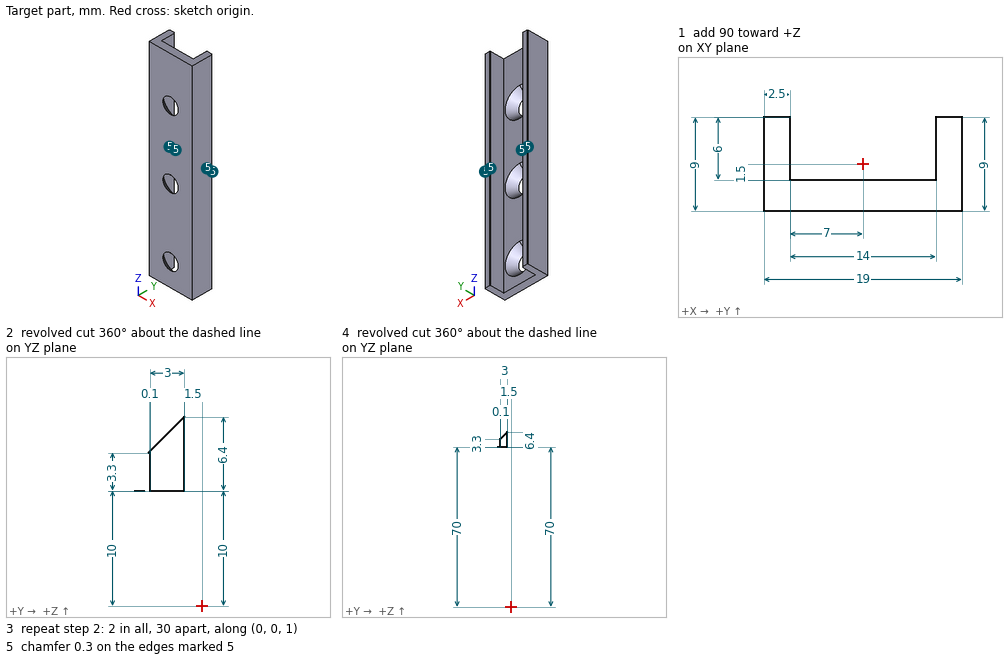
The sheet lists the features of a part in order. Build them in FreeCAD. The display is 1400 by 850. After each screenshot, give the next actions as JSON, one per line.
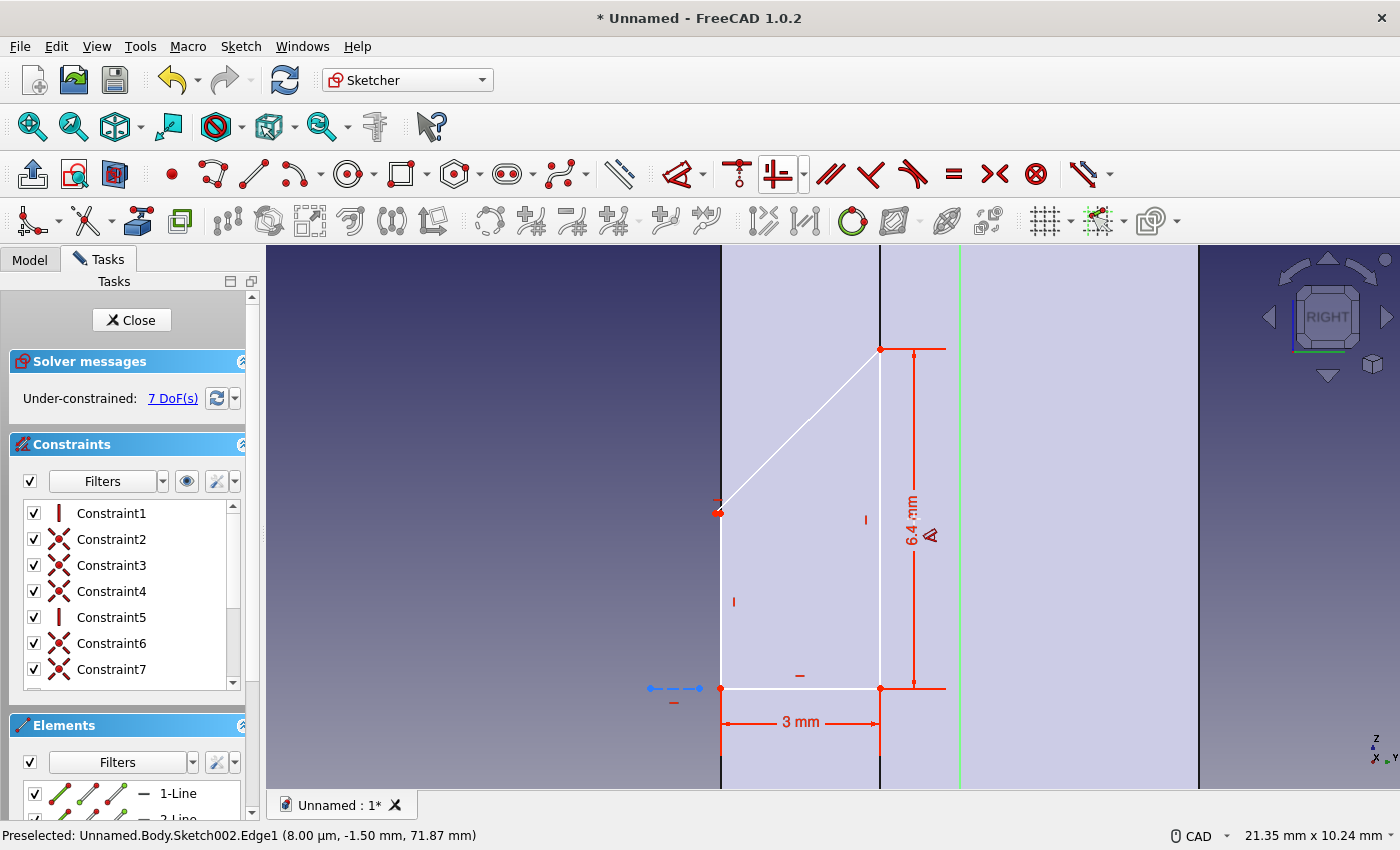
{"action": "scroll", "coordinate": [719, 513], "scroll_direction": "up", "scroll_amount": 11}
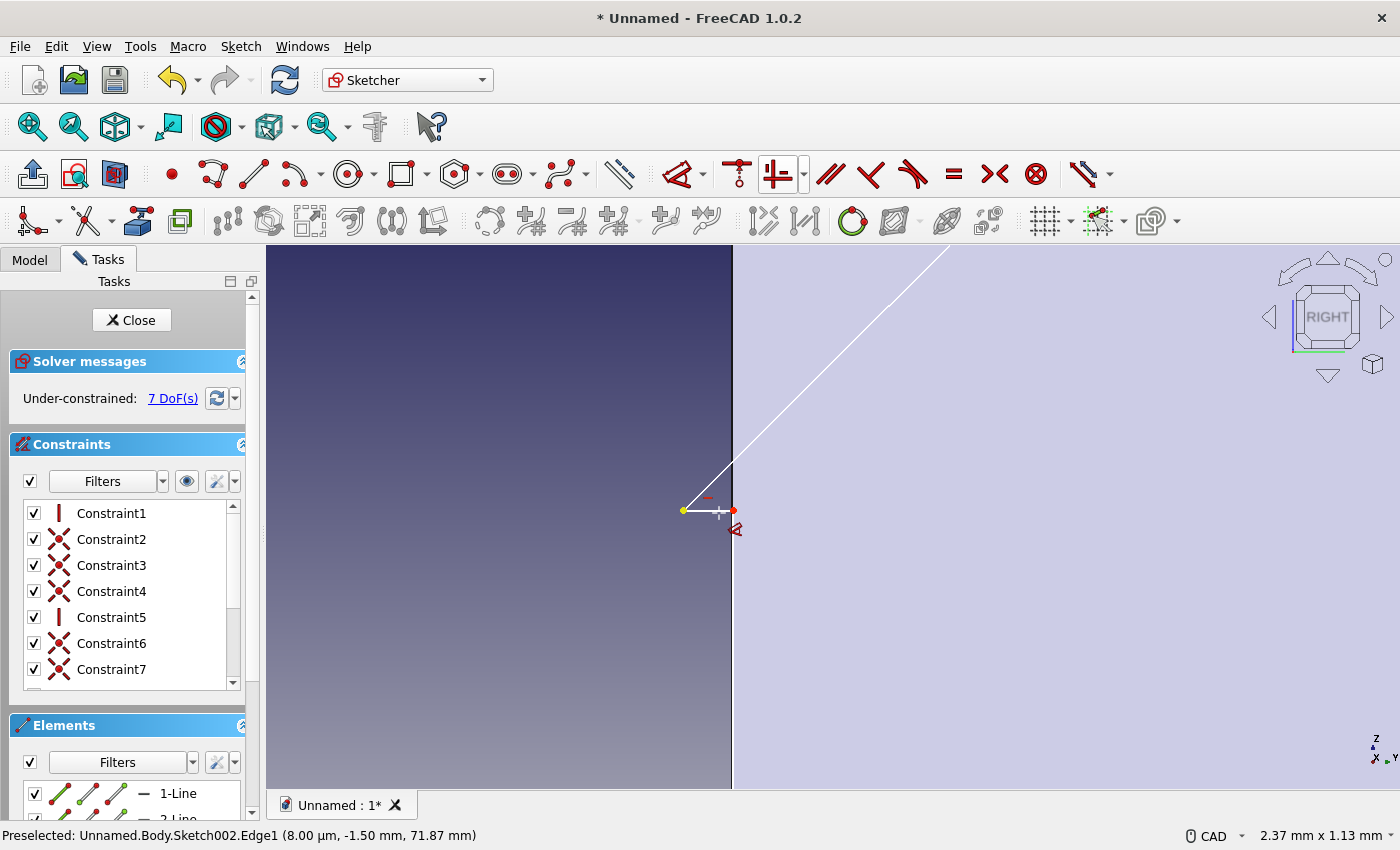
{"action": "left_click", "coordinate": [713, 511]}
{"action": "left_click", "coordinate": [697, 477]}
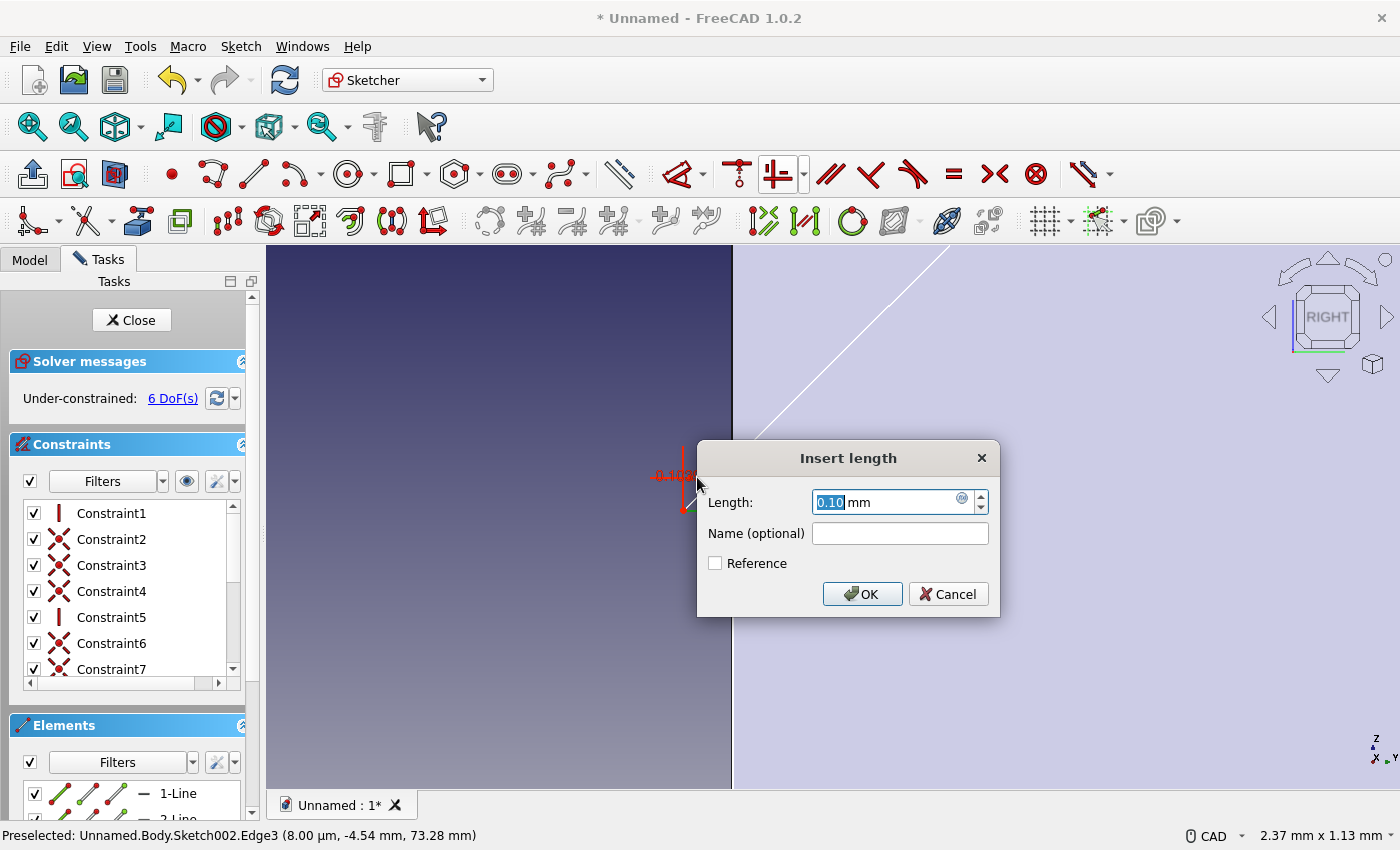
{"action": "type", "text": "0.1"}
{"action": "key", "text": "Return"}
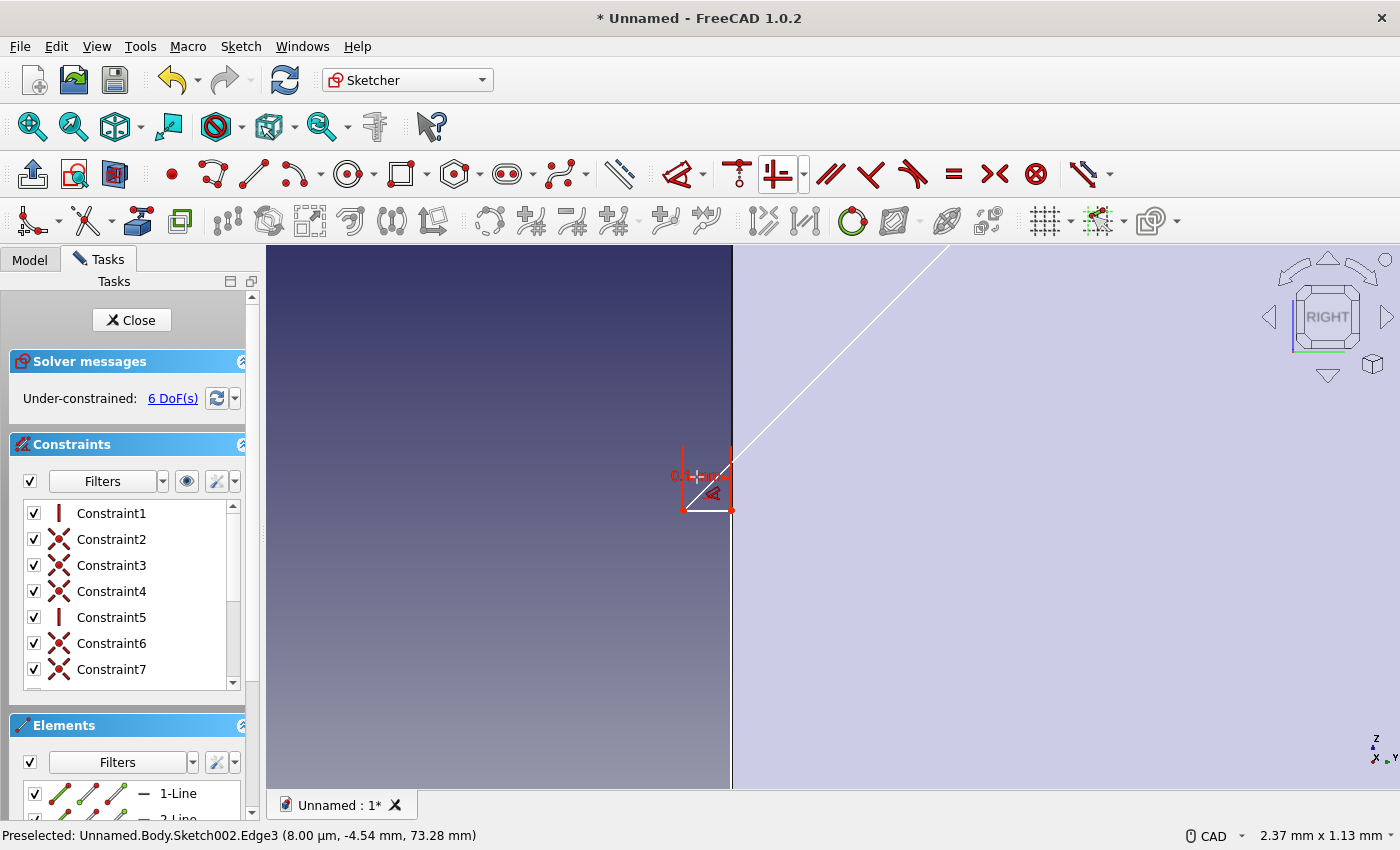
{"action": "scroll", "coordinate": [719, 513], "scroll_direction": "down", "scroll_amount": 11}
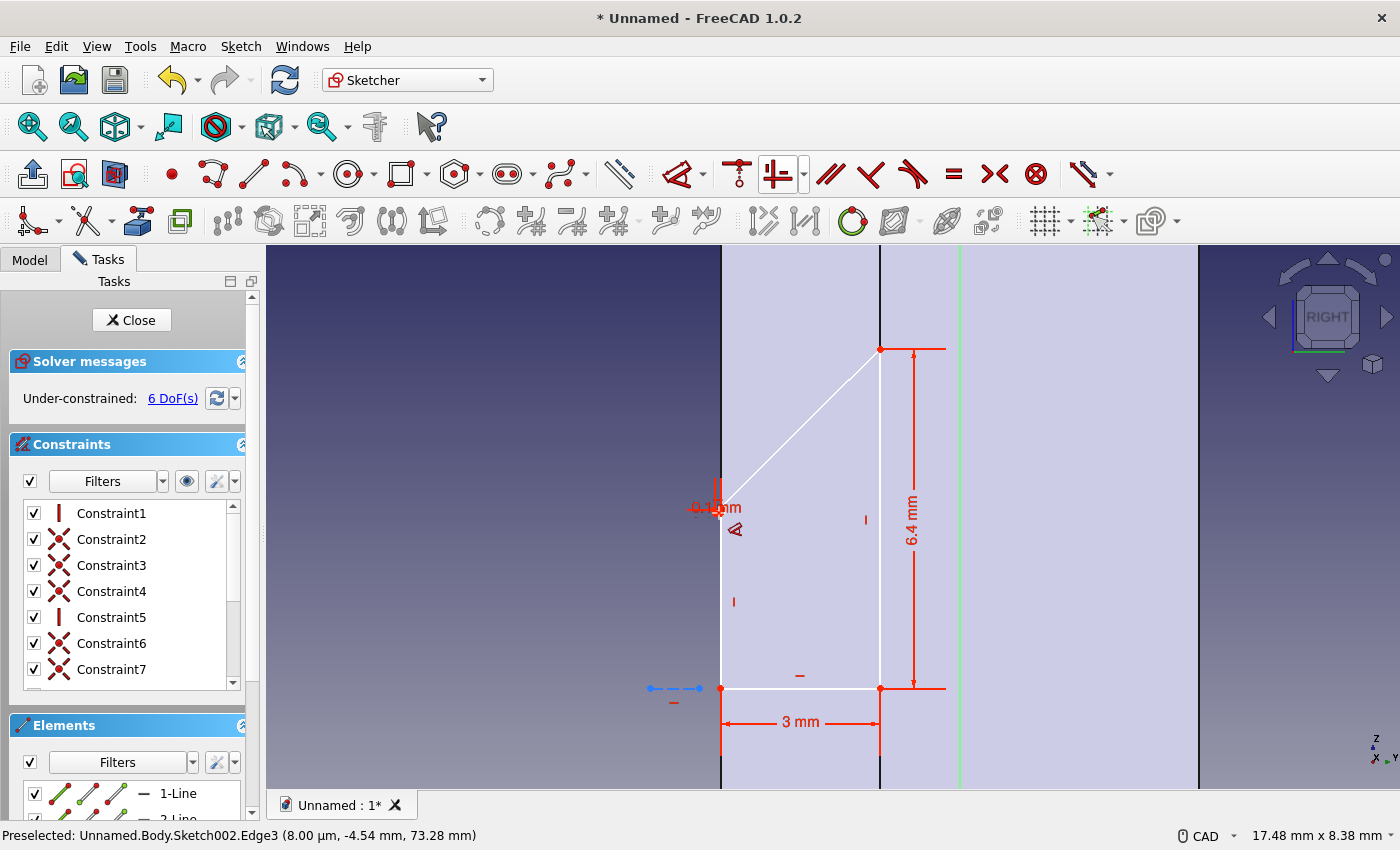
{"action": "left_click", "coordinate": [721, 566]}
{"action": "left_click", "coordinate": [687, 601]}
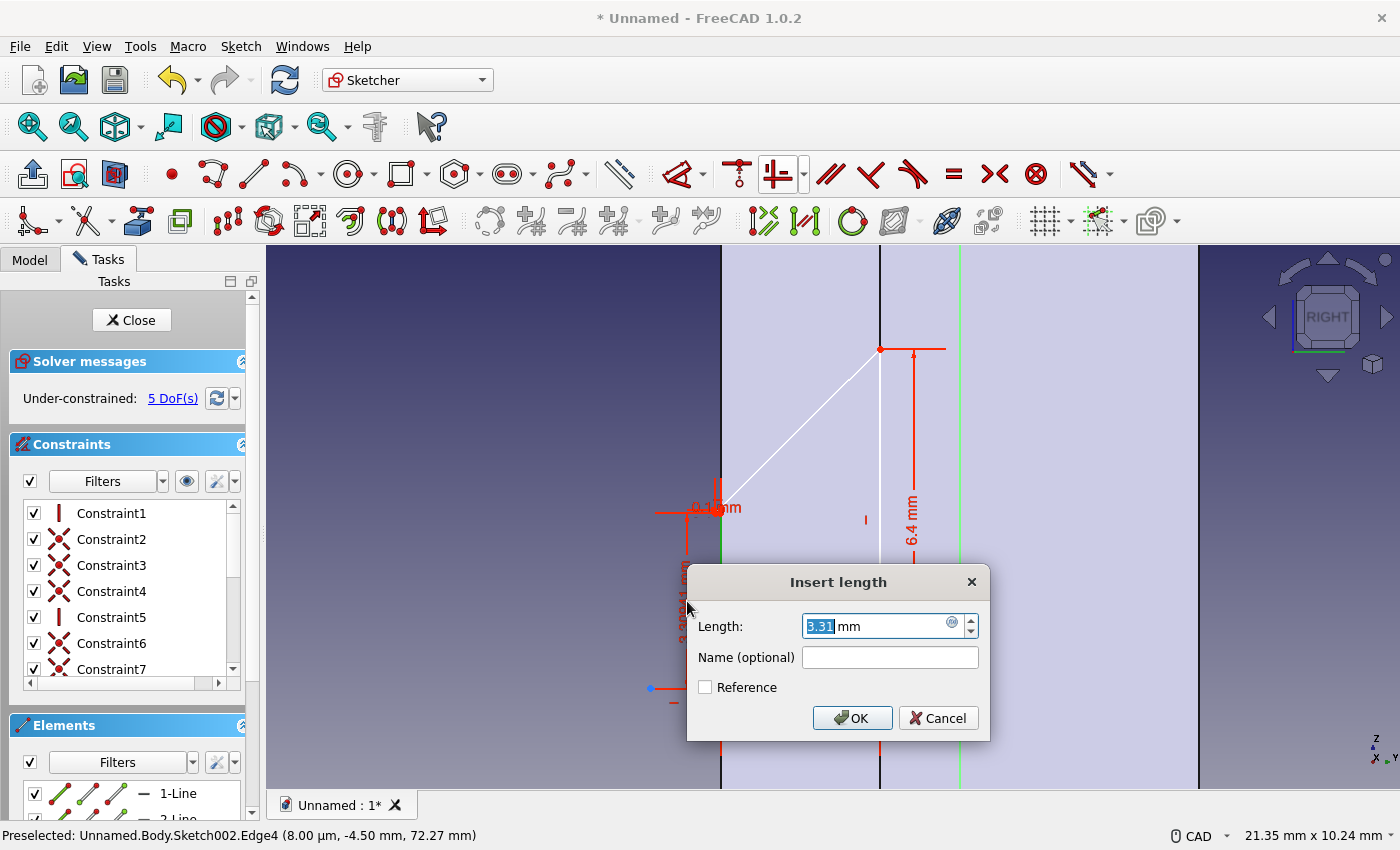
{"action": "type", "text": "3.3"}
{"action": "key", "text": "Return"}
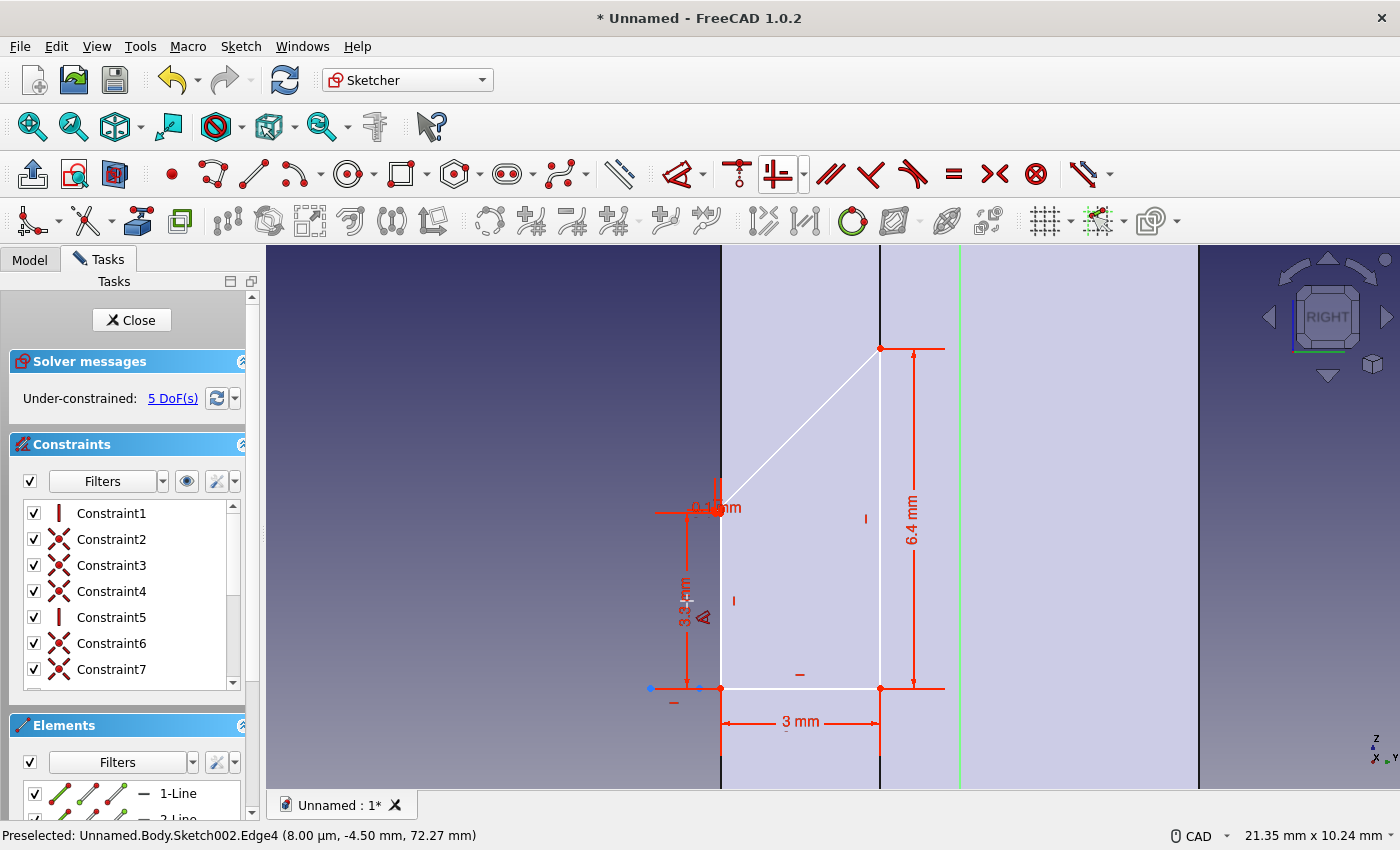
{"action": "left_click", "coordinate": [880, 688]}
{"action": "left_click", "coordinate": [994, 725]}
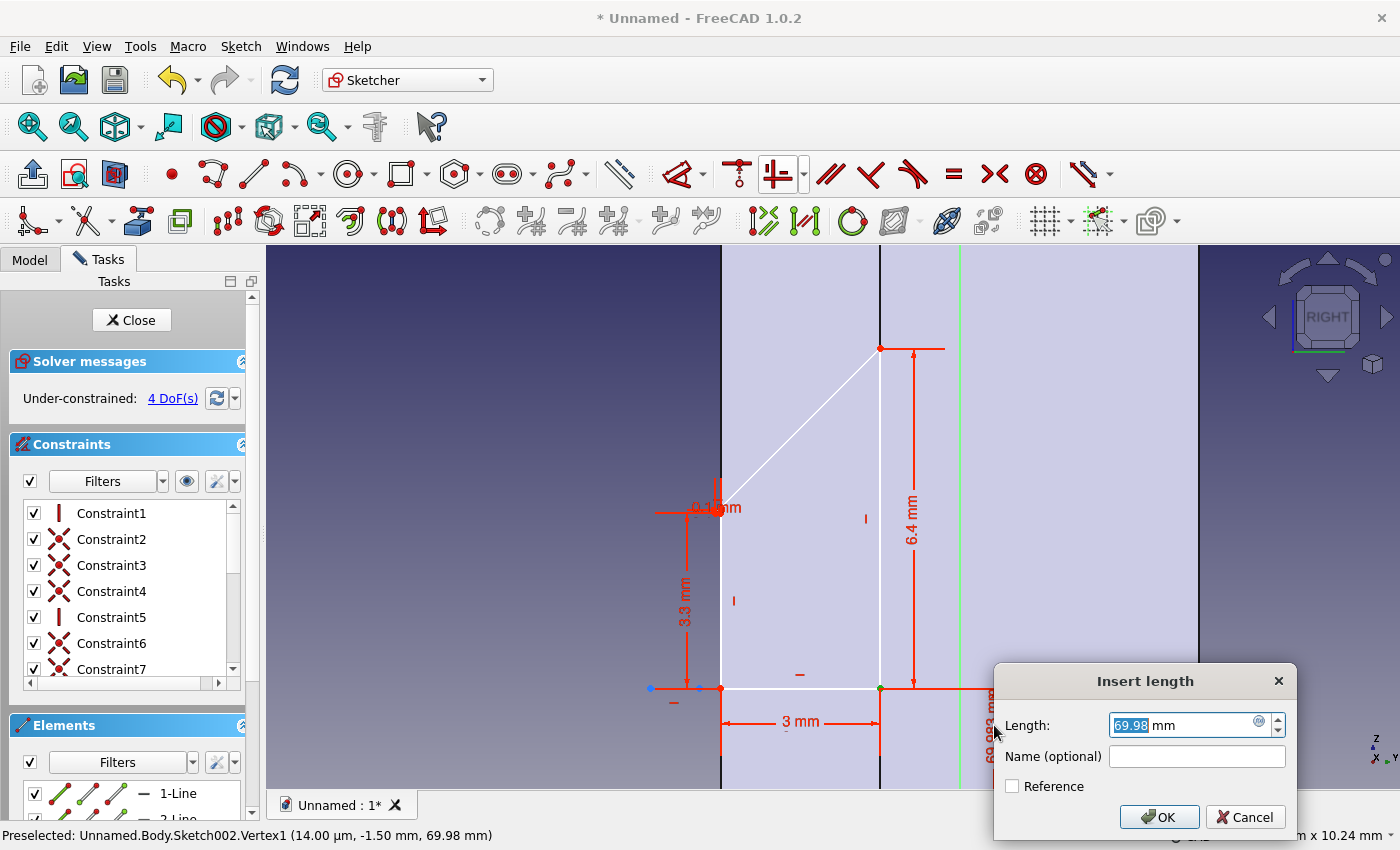
{"action": "type", "text": "70"}
{"action": "key", "text": "Return"}